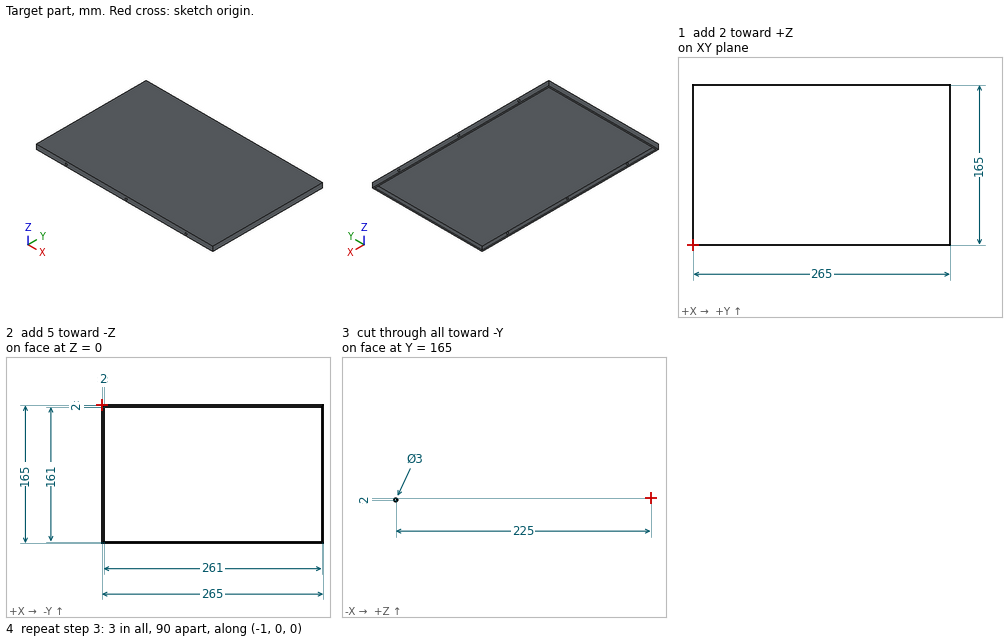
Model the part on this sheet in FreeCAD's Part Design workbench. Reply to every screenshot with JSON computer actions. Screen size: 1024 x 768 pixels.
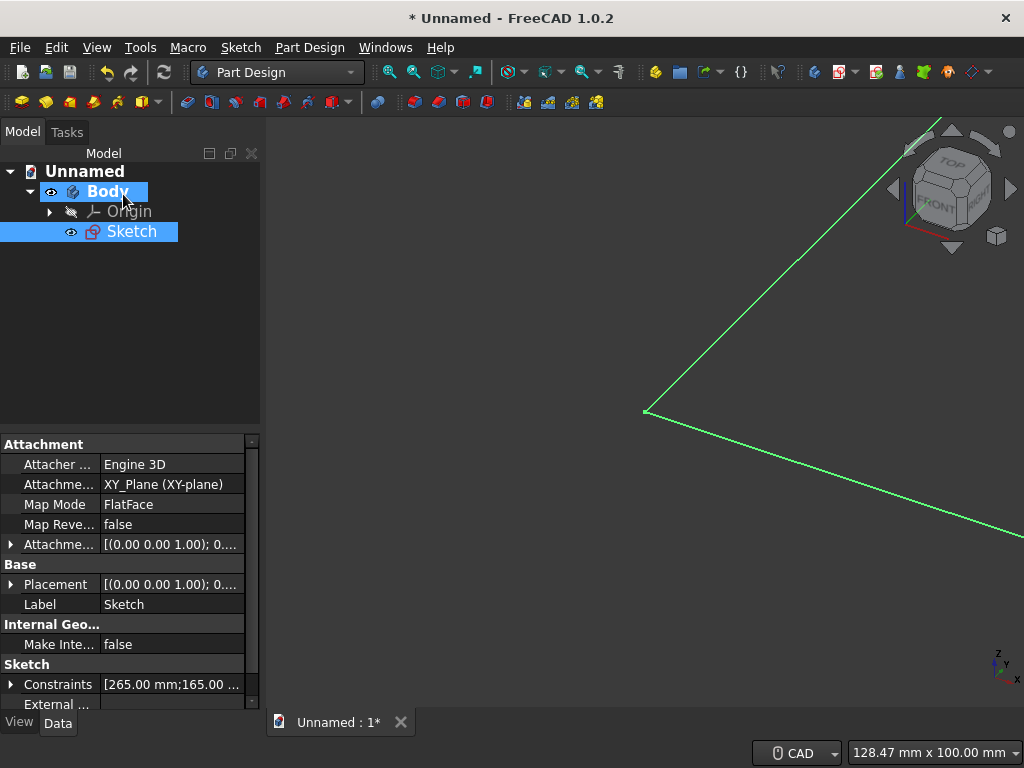
{"action": "left_click", "coordinate": [22, 102]}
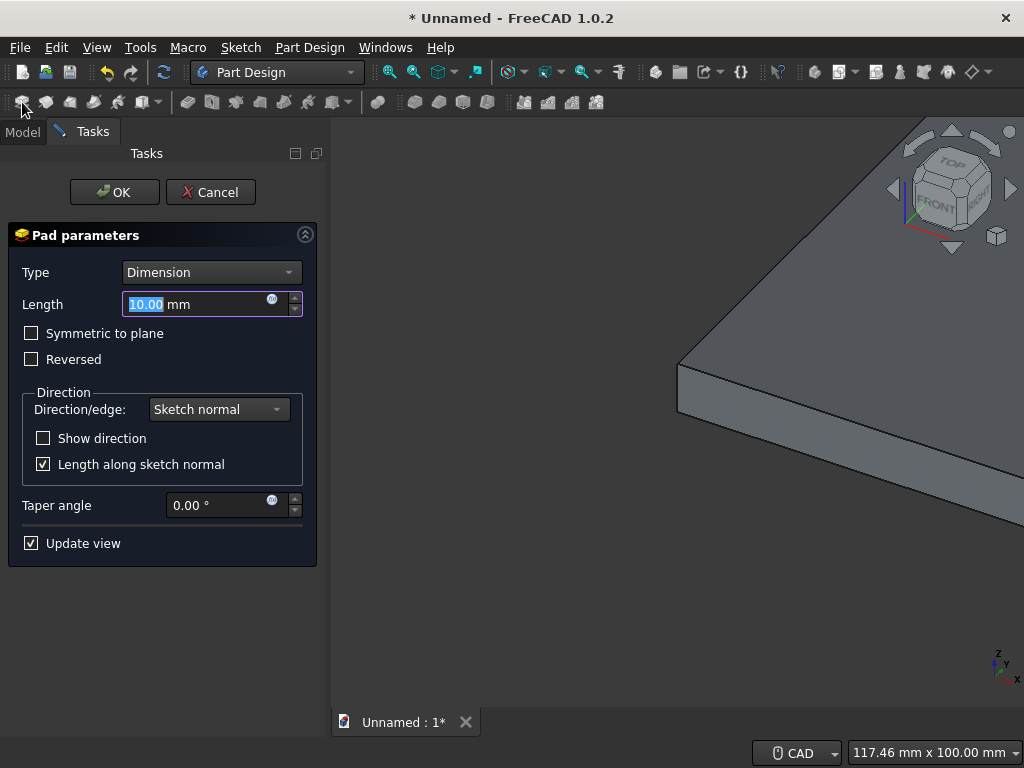
{"action": "type", "text": "2"}
{"action": "key", "text": "Tab"}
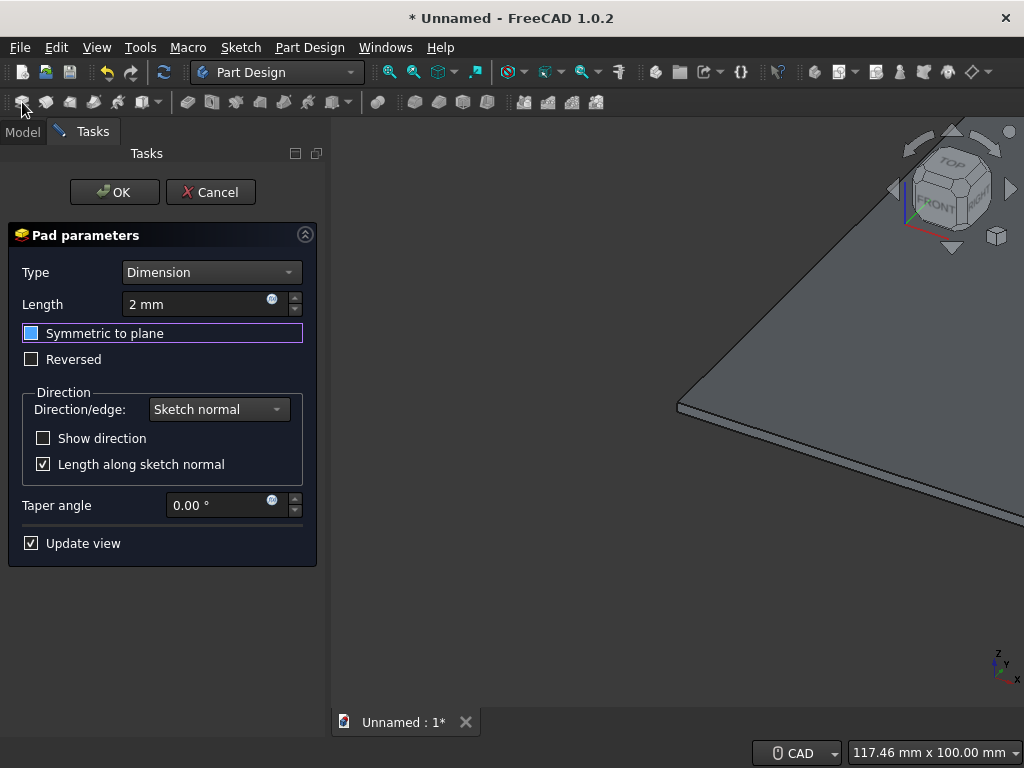
{"action": "left_click", "coordinate": [115, 192]}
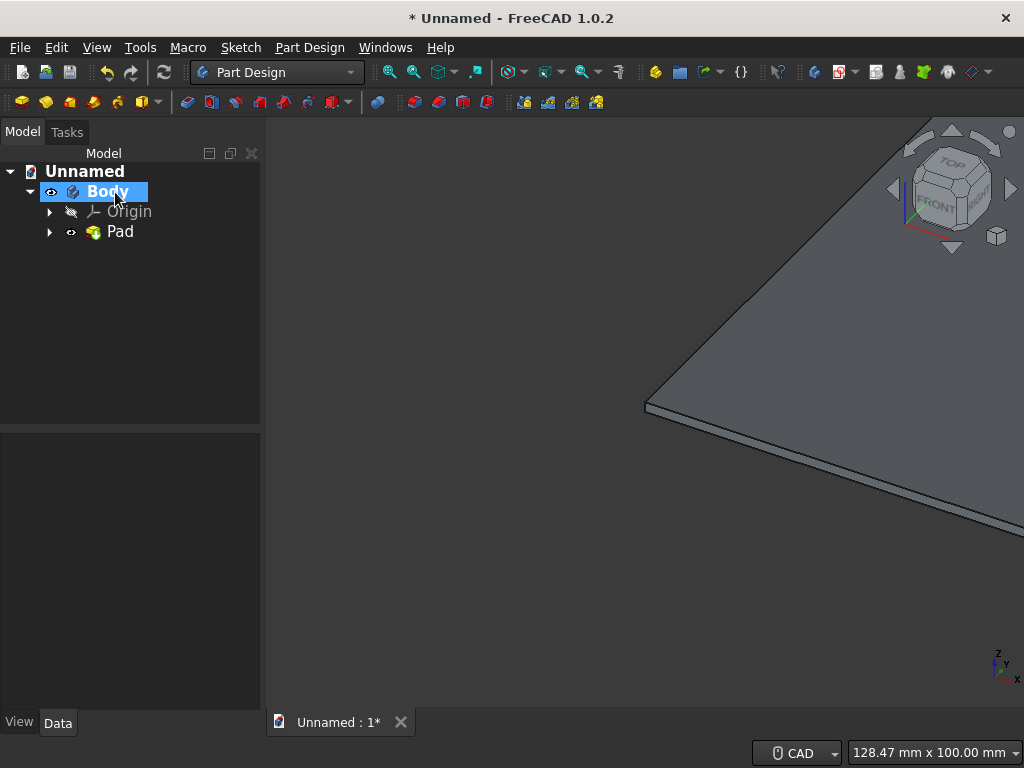
{"action": "key", "text": "v f"}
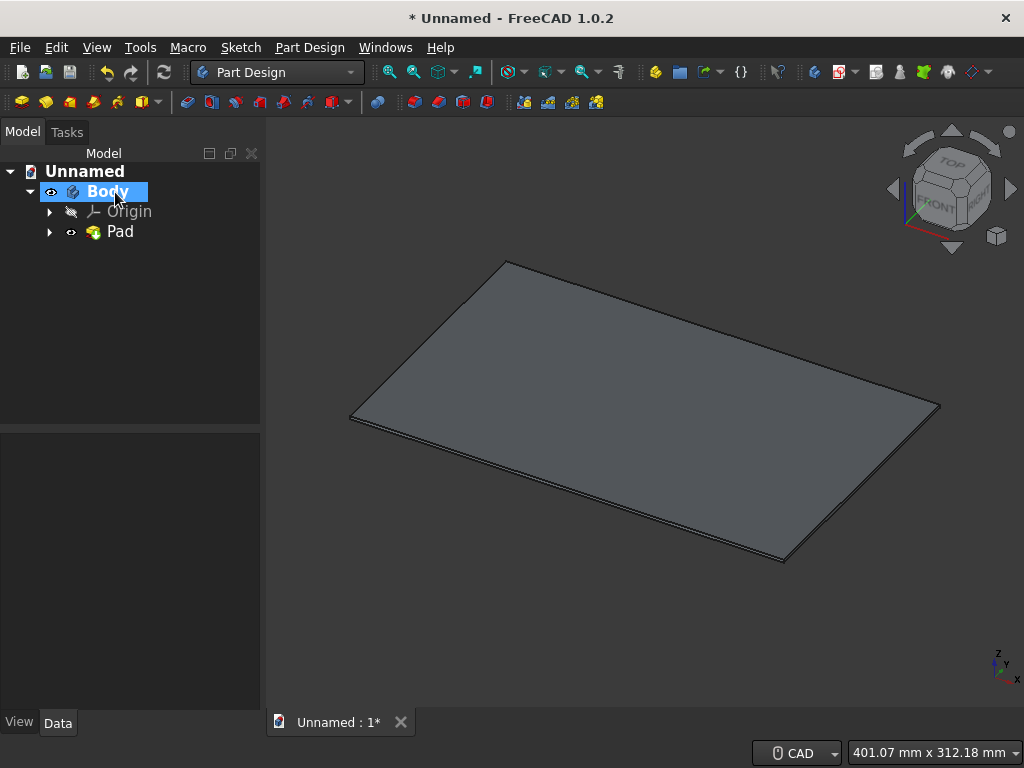
{"action": "key", "text": "5"}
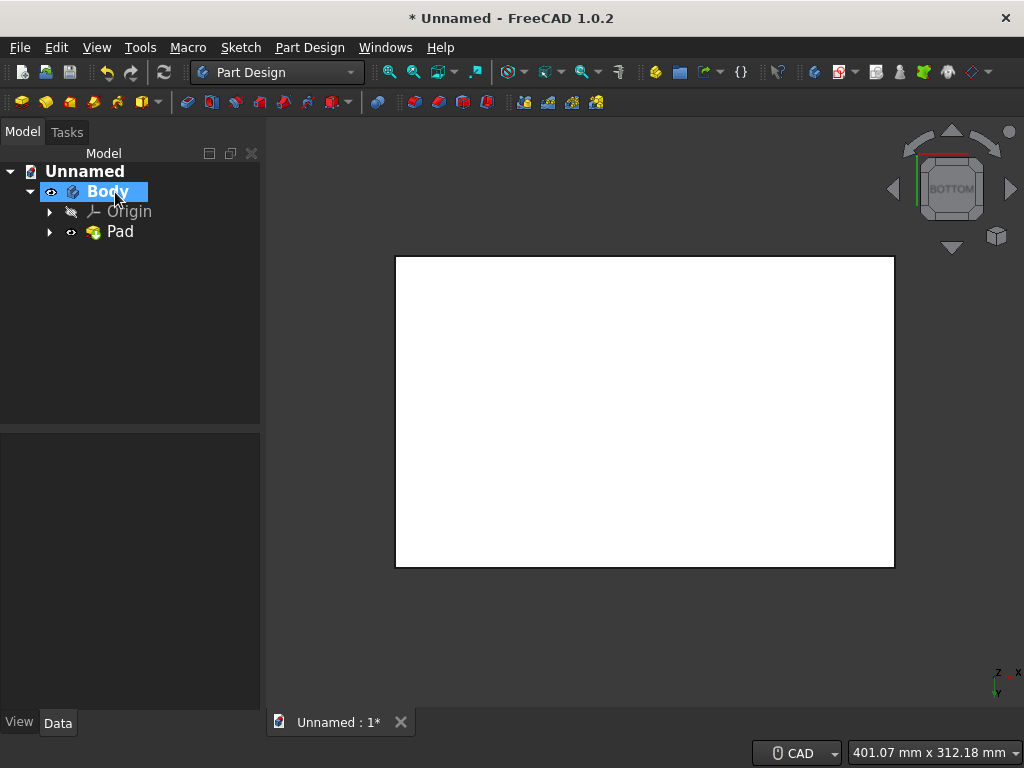
{"action": "left_click", "coordinate": [717, 411]}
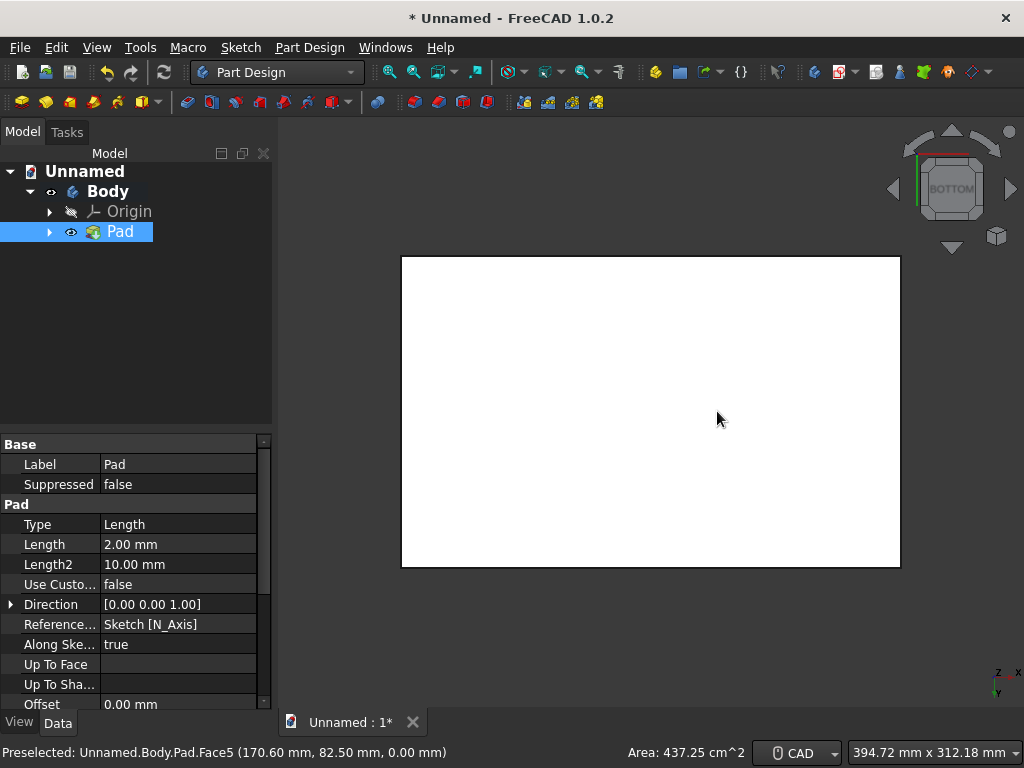
{"action": "left_click", "coordinate": [840, 72]}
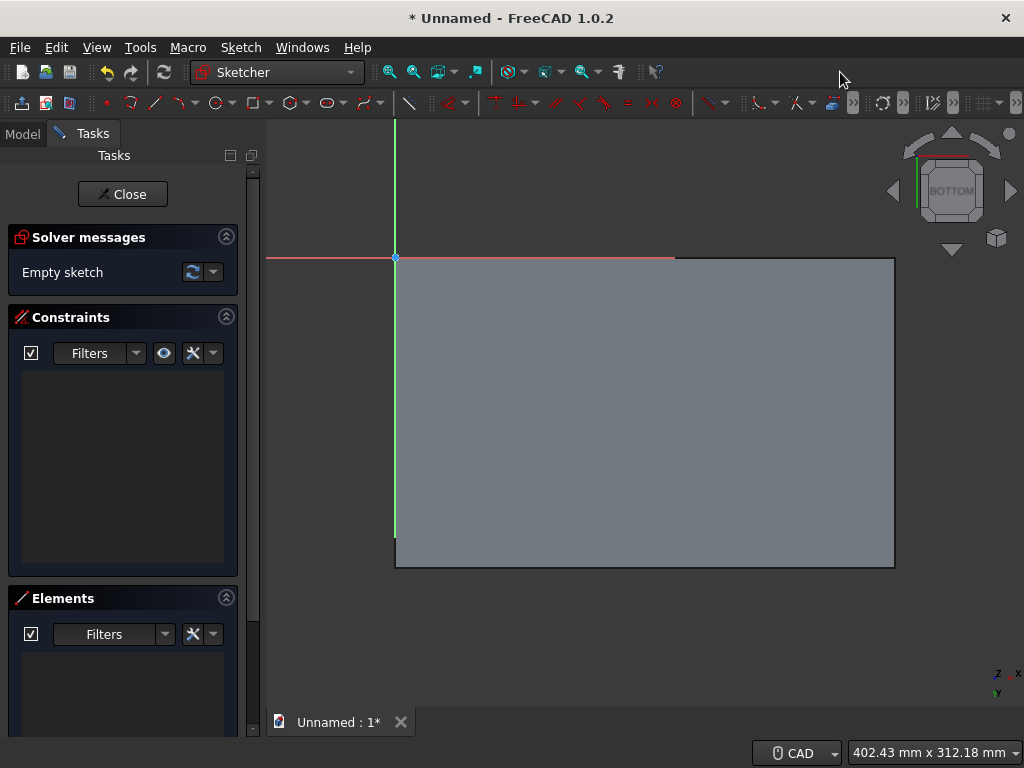
{"action": "scroll", "coordinate": [294, 413], "scroll_direction": "down", "scroll_amount": 1}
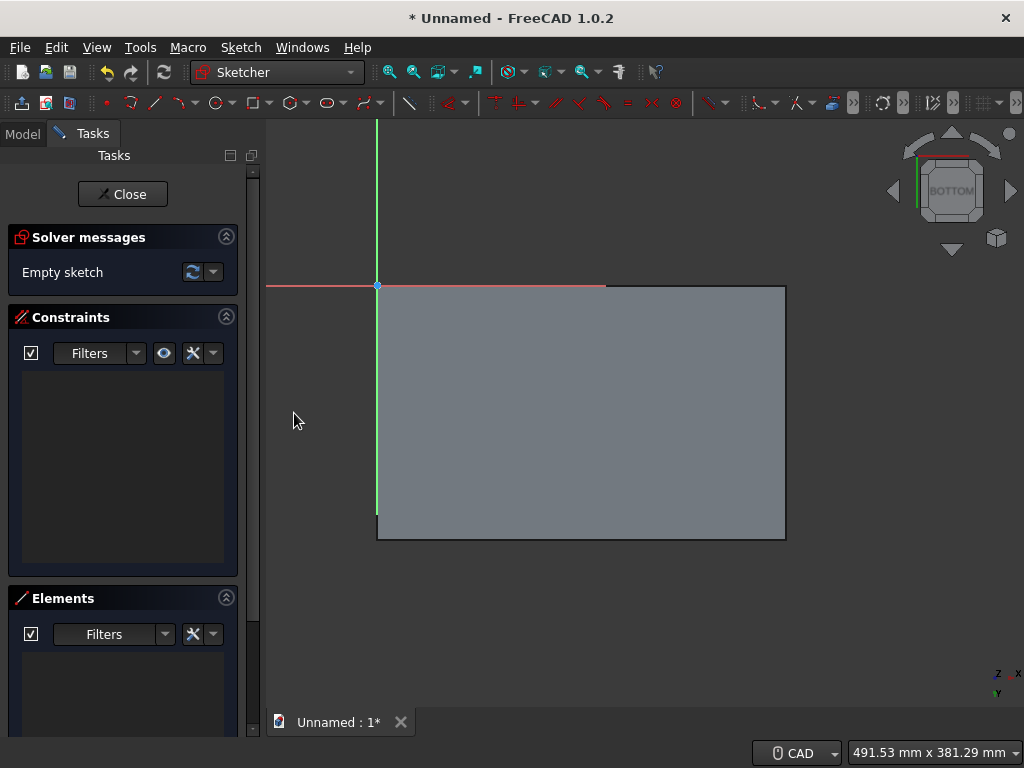
{"action": "left_click", "coordinate": [254, 104]}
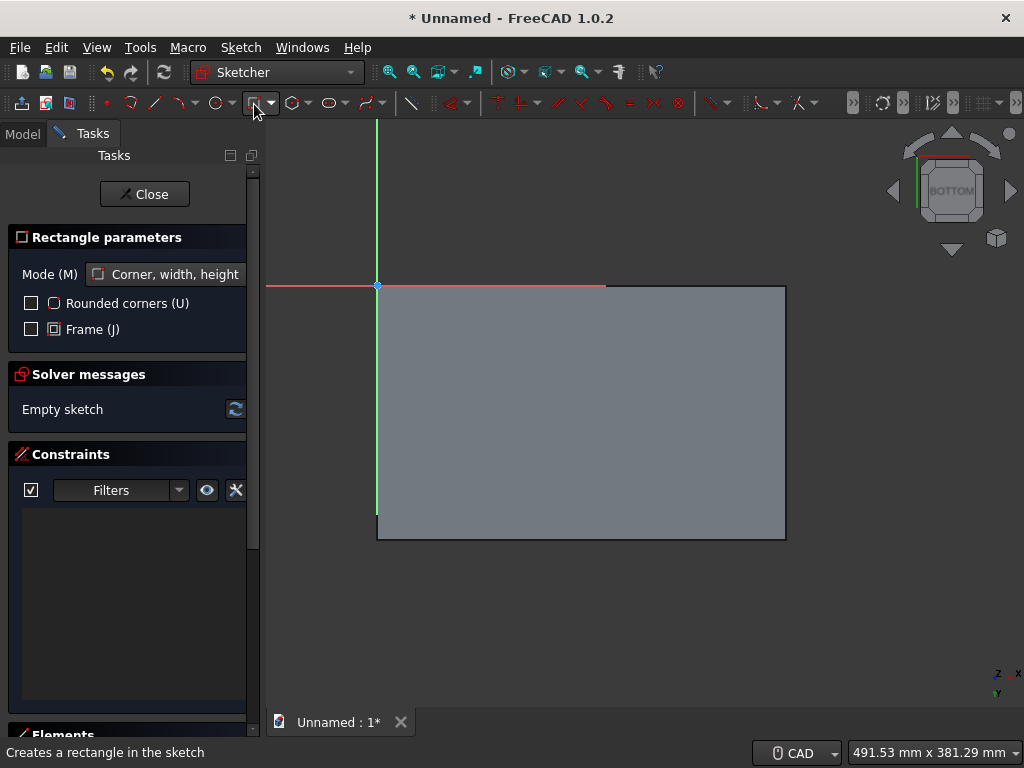
{"action": "left_click", "coordinate": [377, 286]}
{"action": "left_click", "coordinate": [786, 540]}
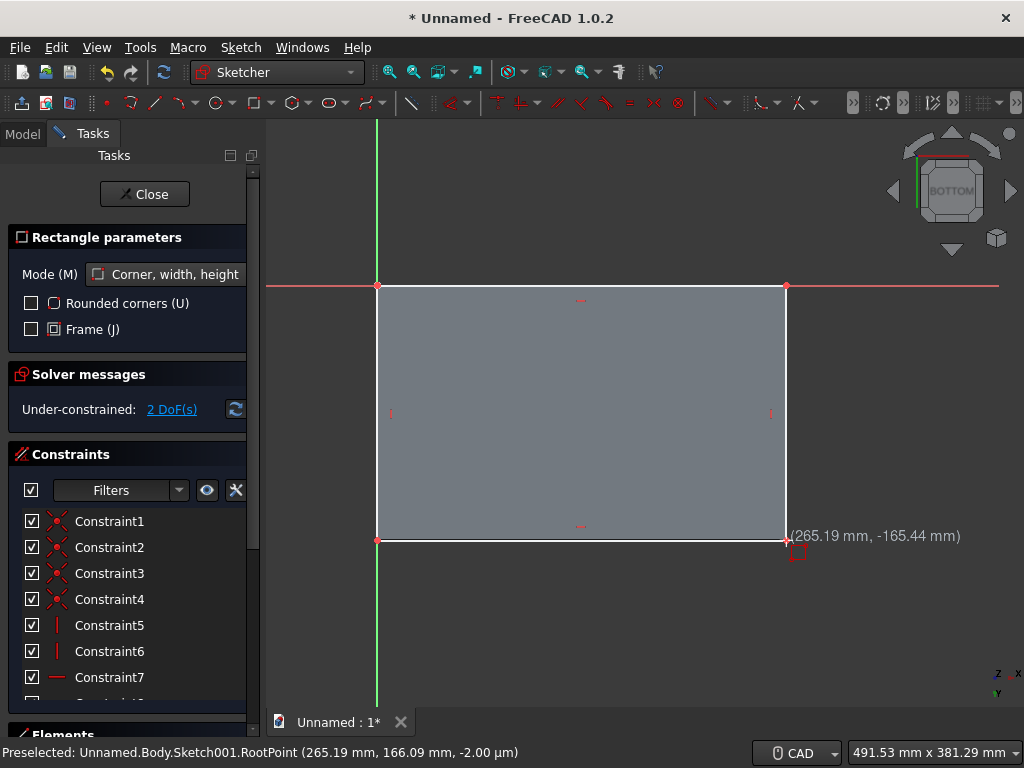
{"action": "scroll", "coordinate": [380, 289], "scroll_direction": "up", "scroll_amount": 9}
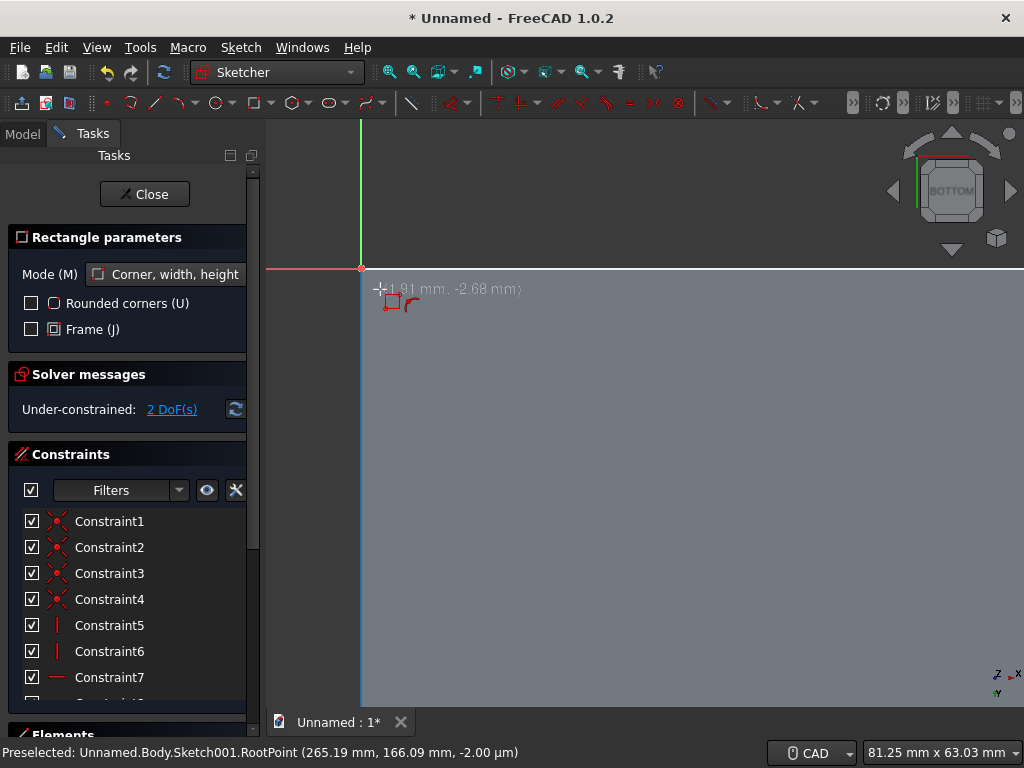
{"action": "left_click", "coordinate": [380, 287]}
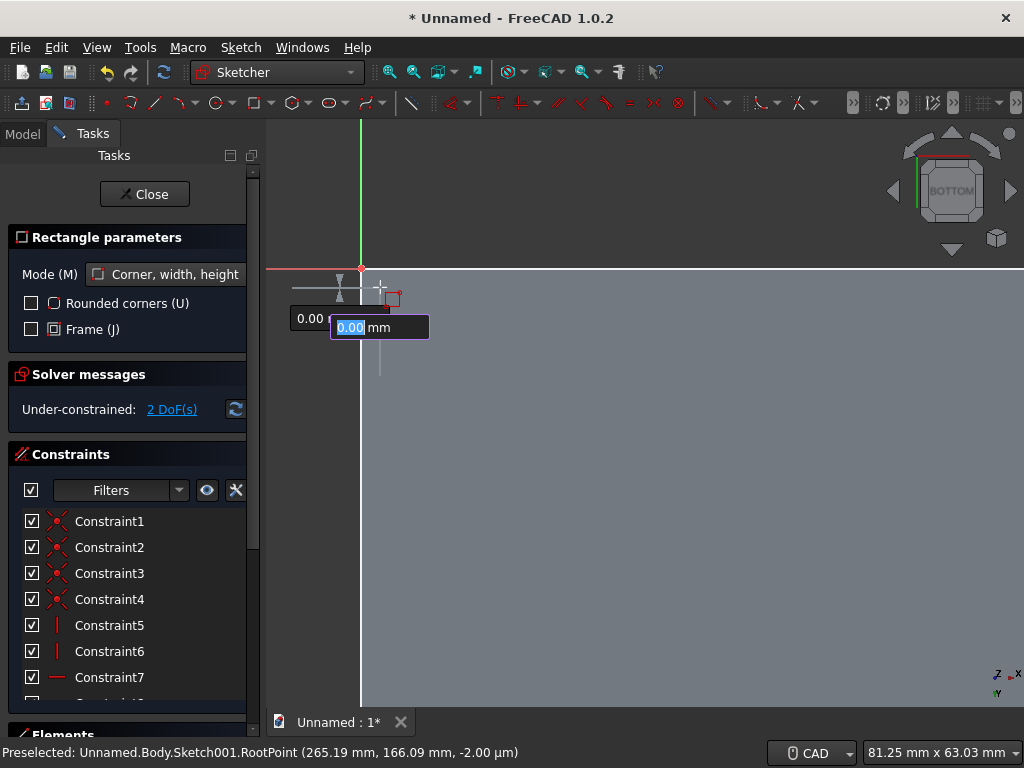
{"action": "scroll", "coordinate": [374, 289], "scroll_direction": "down", "scroll_amount": 9}